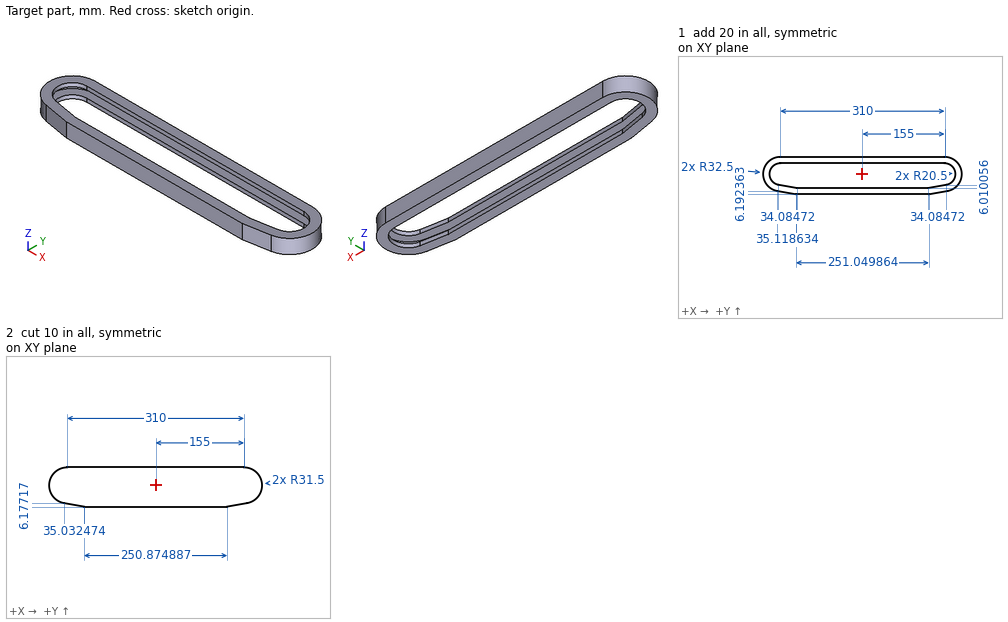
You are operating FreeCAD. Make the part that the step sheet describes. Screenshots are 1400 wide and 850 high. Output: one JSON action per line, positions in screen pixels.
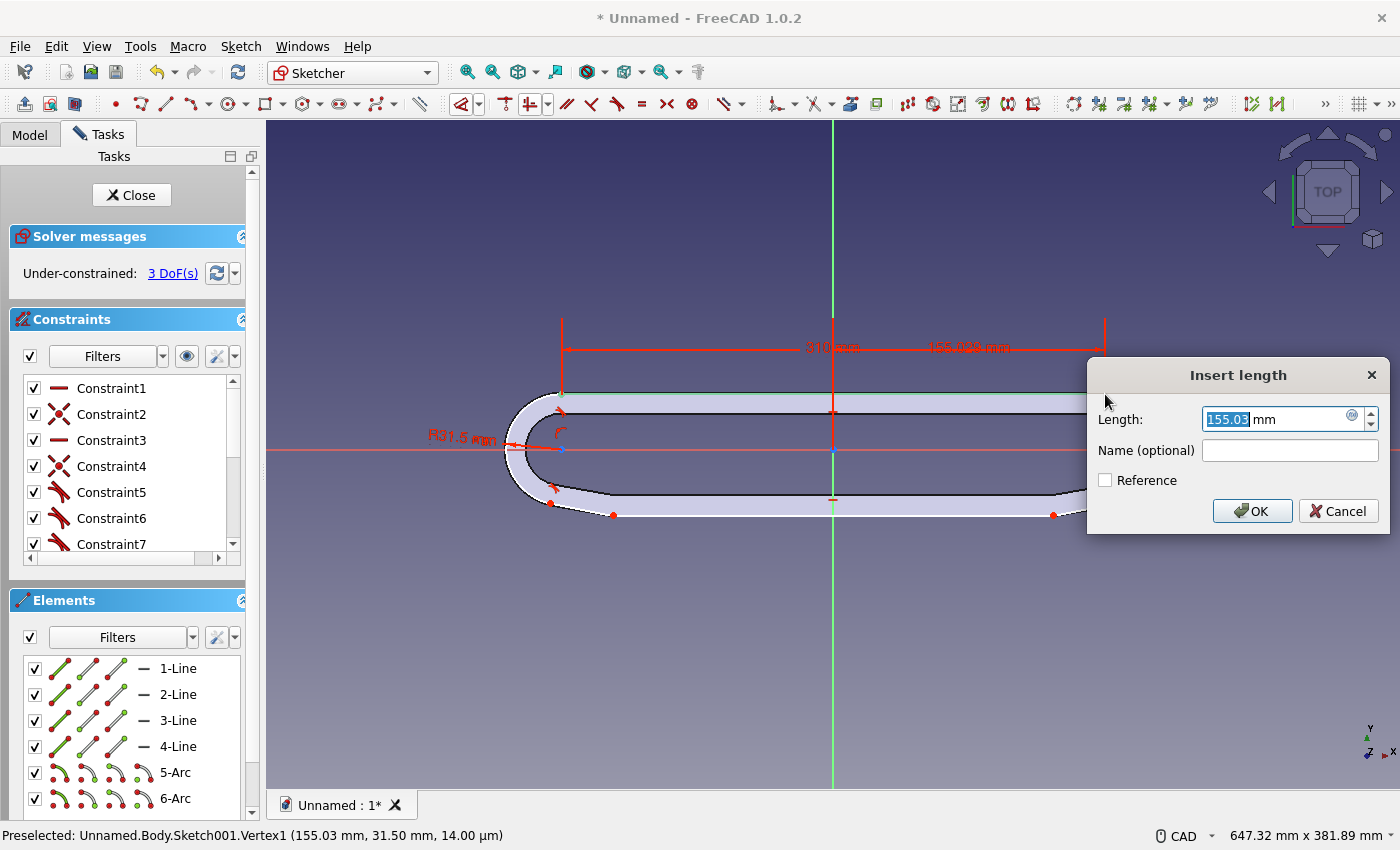
{"action": "type", "text": "155"}
{"action": "key", "text": "Return"}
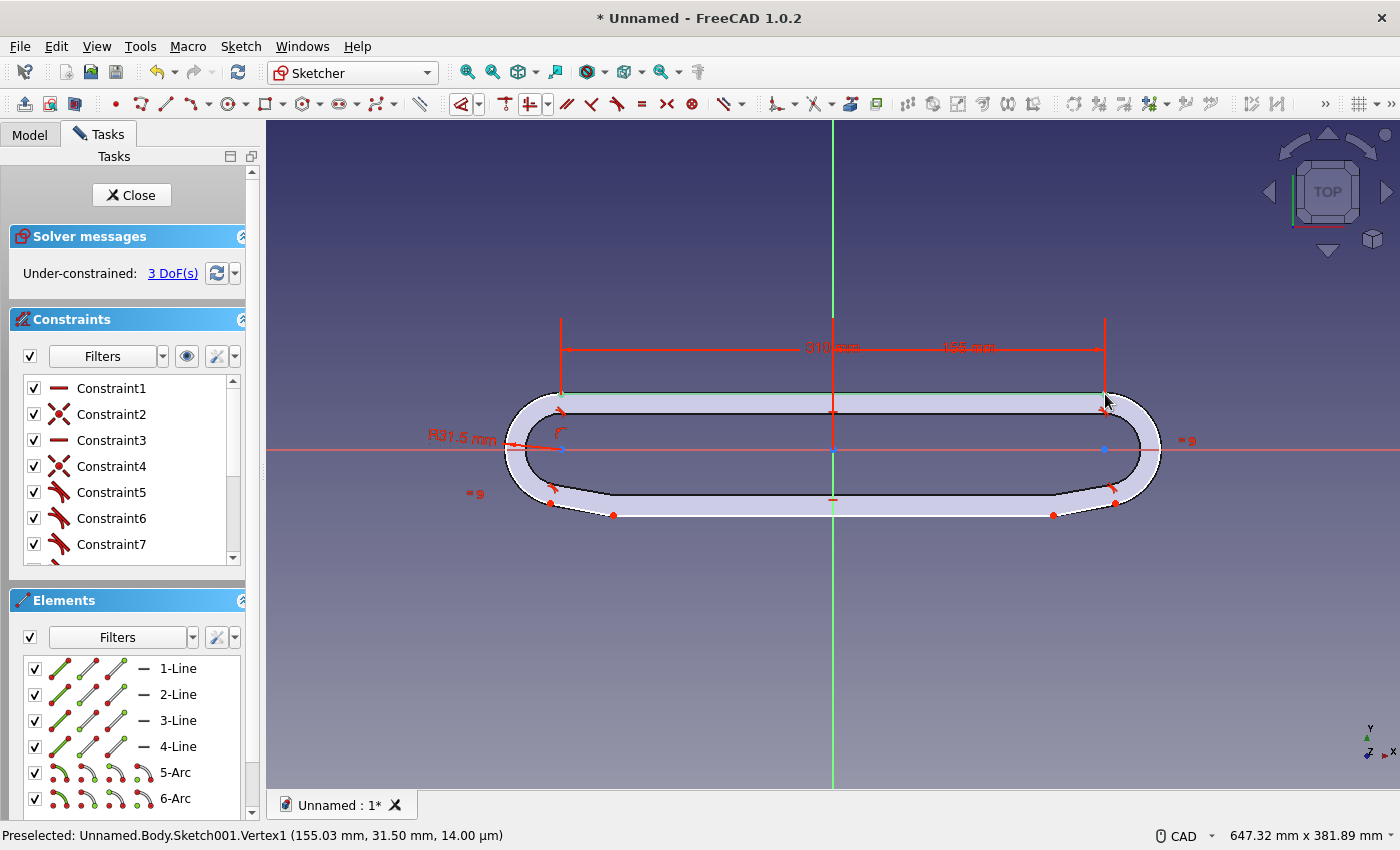
{"action": "scroll", "coordinate": [569, 507], "scroll_direction": "up", "scroll_amount": 7}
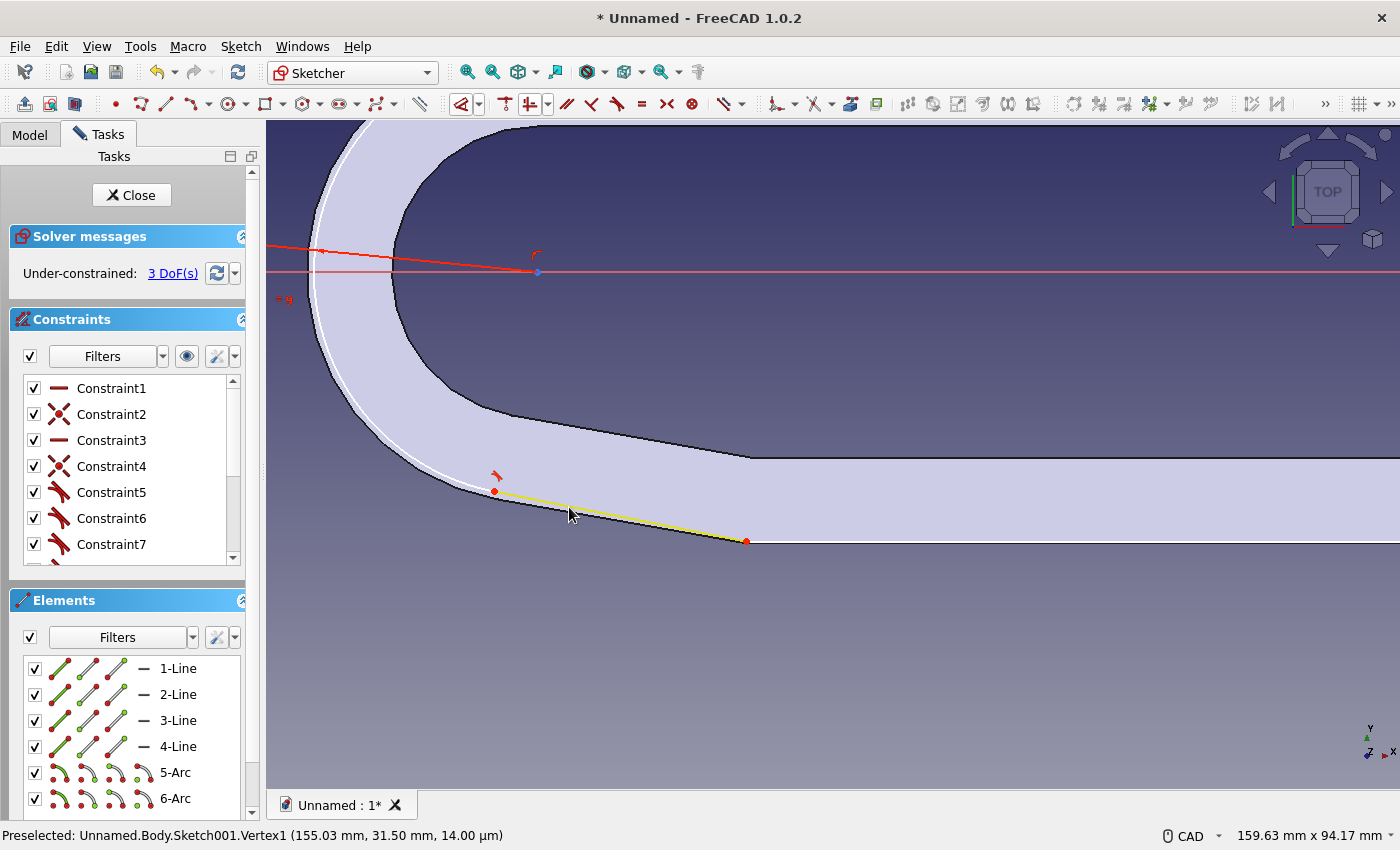
{"action": "left_click", "coordinate": [570, 507]}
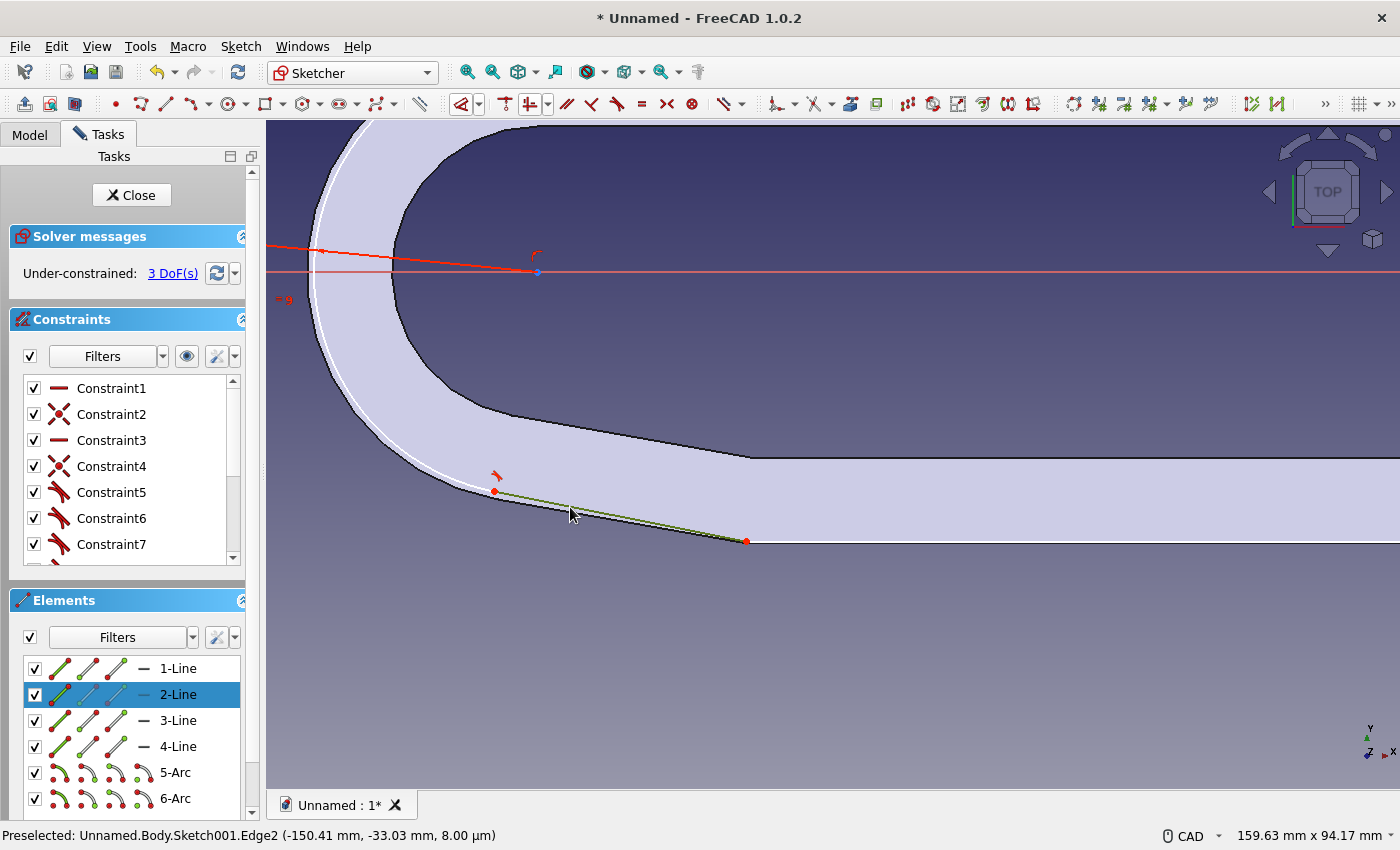
{"action": "key", "text": "i"}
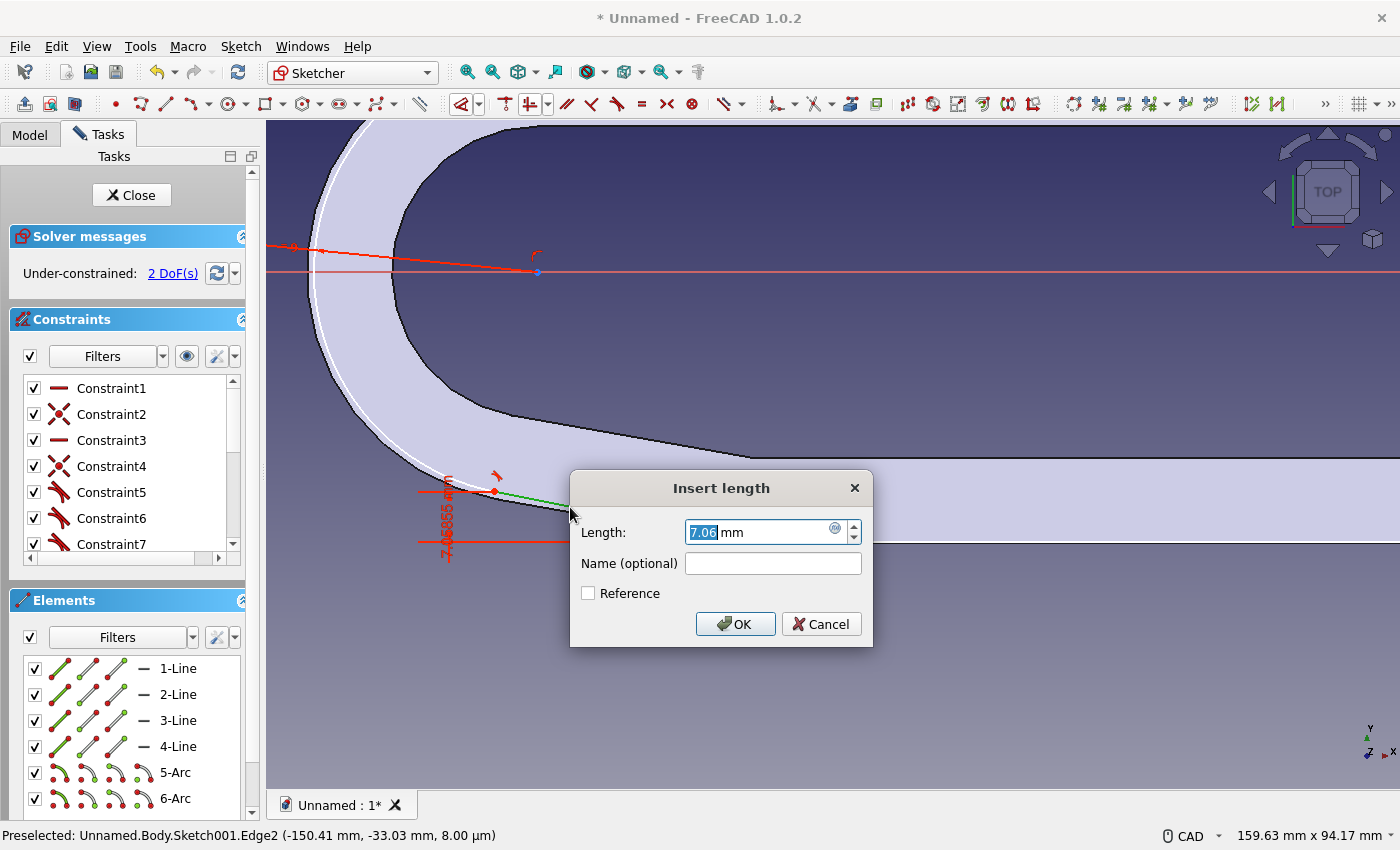
{"action": "type", "text": "6.17717"}
{"action": "key", "text": "Return"}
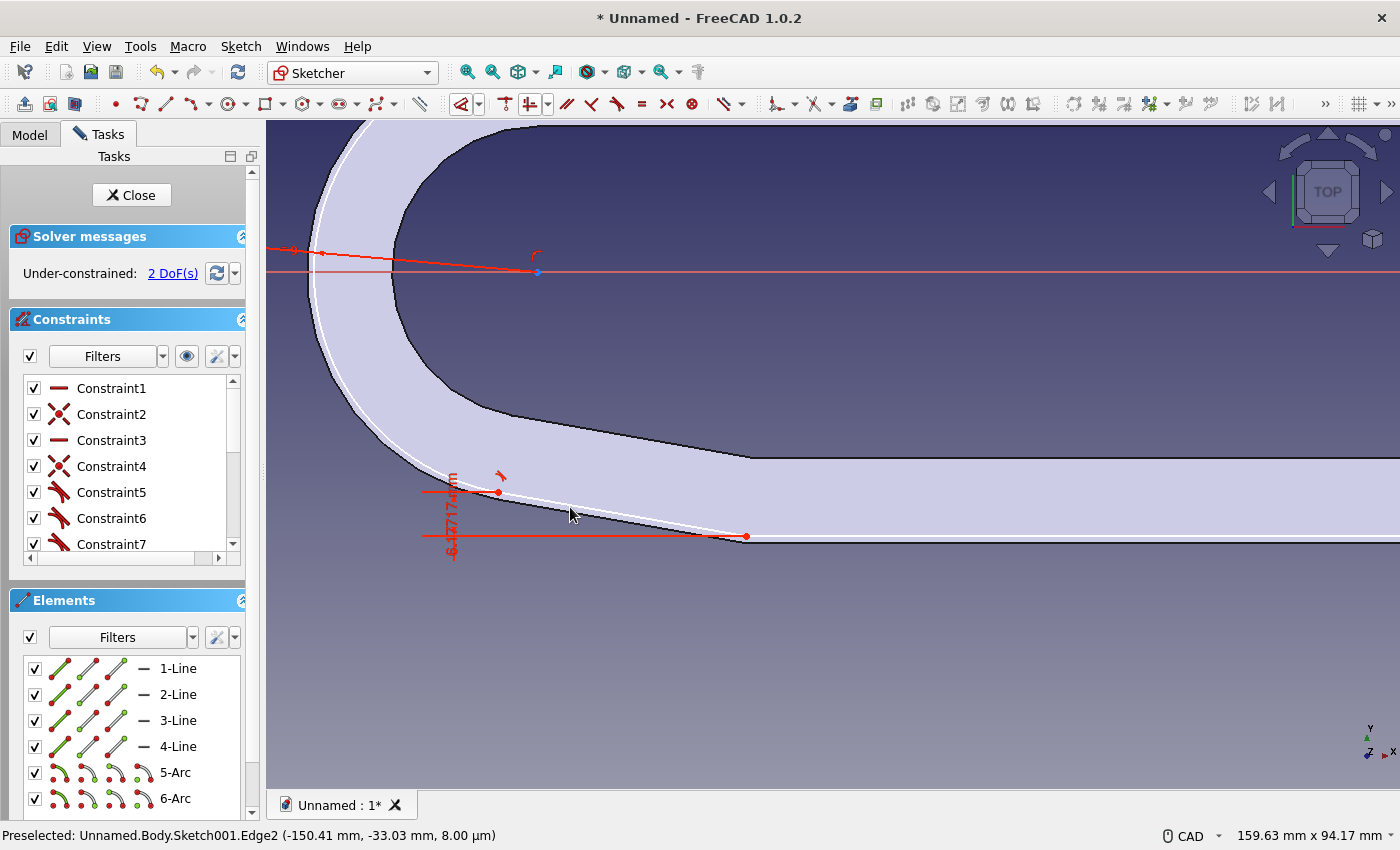
{"action": "scroll", "coordinate": [478, 508], "scroll_direction": "down", "scroll_amount": 7}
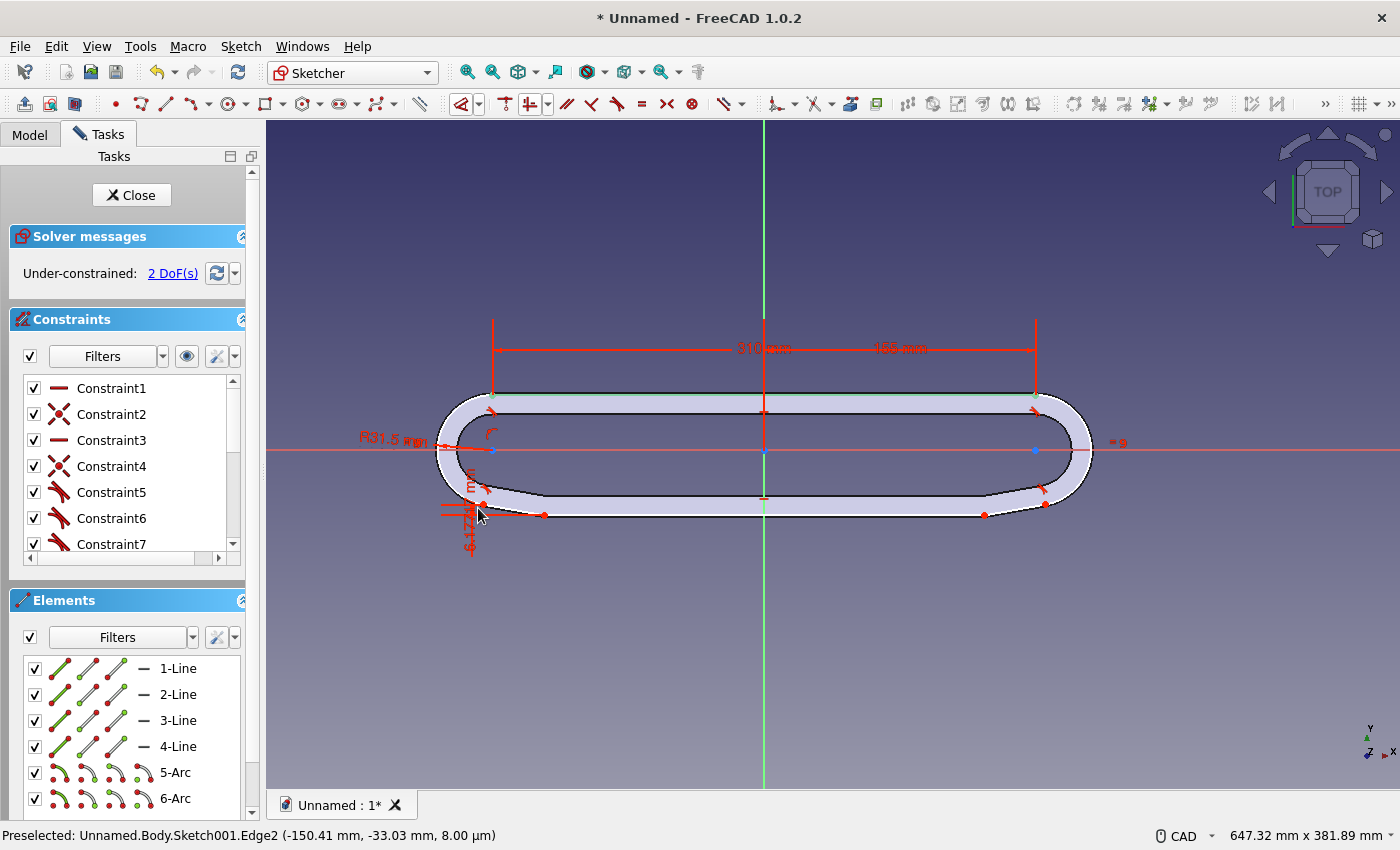
{"action": "left_click", "coordinate": [632, 515]}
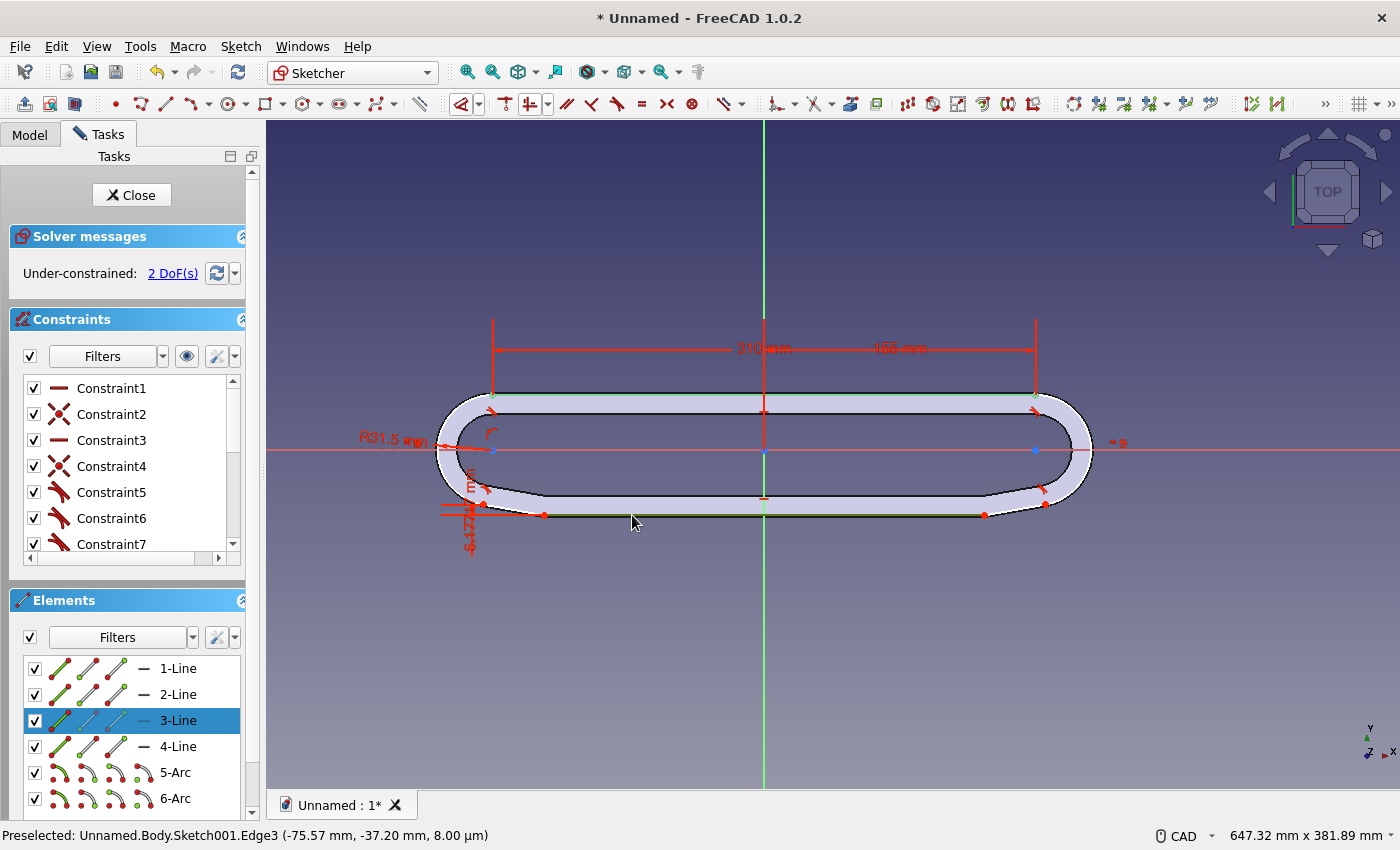
{"action": "left_click", "coordinate": [478, 104]}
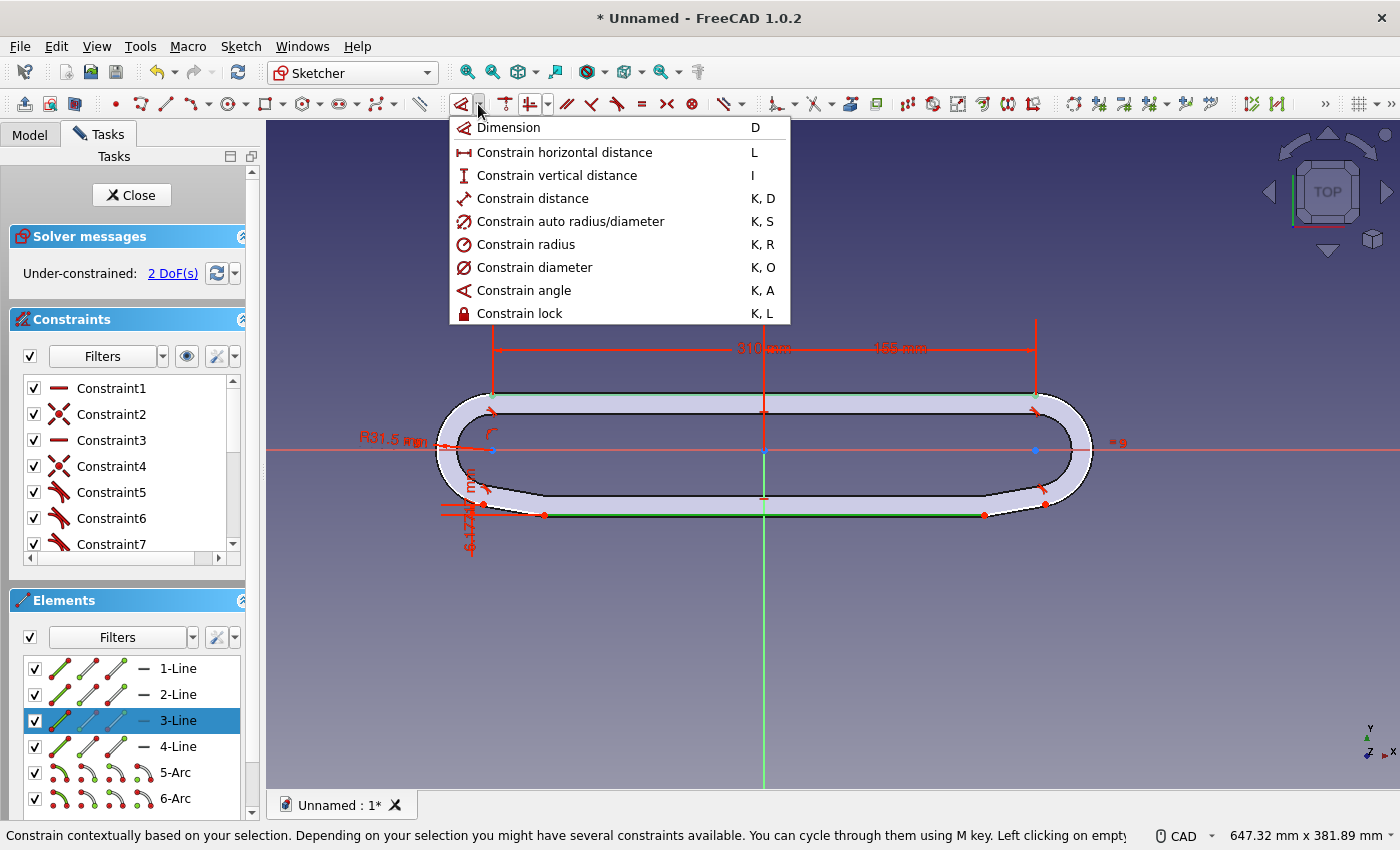
{"action": "left_click", "coordinate": [620, 152]}